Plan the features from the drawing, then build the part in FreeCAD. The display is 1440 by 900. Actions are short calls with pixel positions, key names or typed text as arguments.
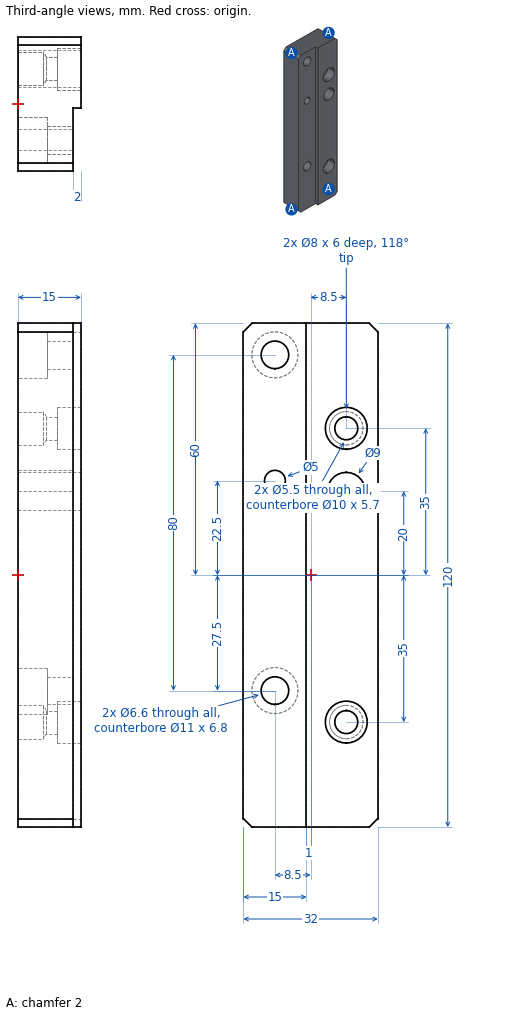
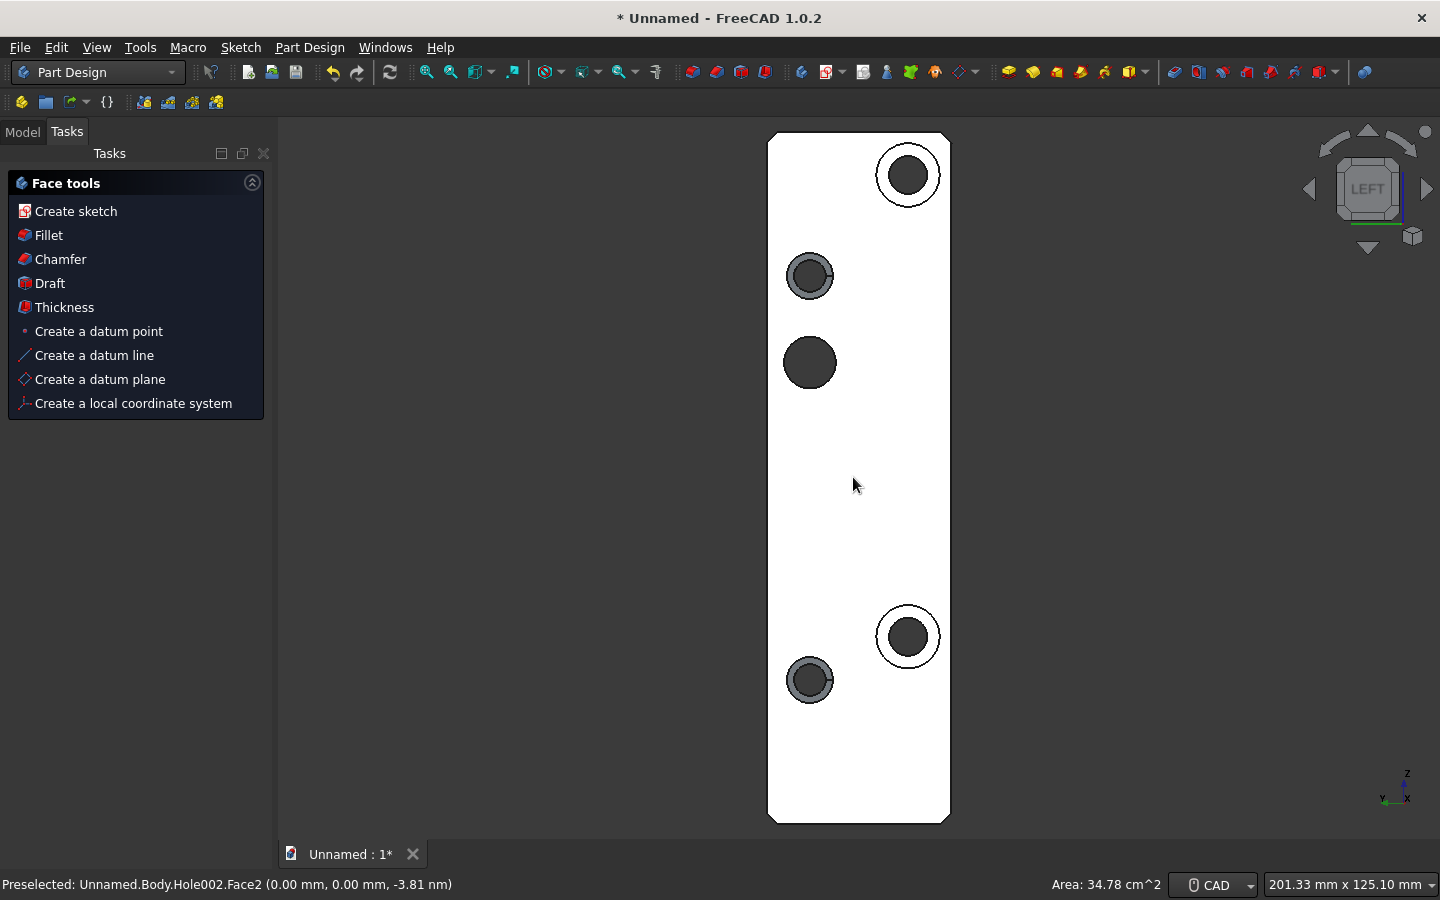
click(826, 72)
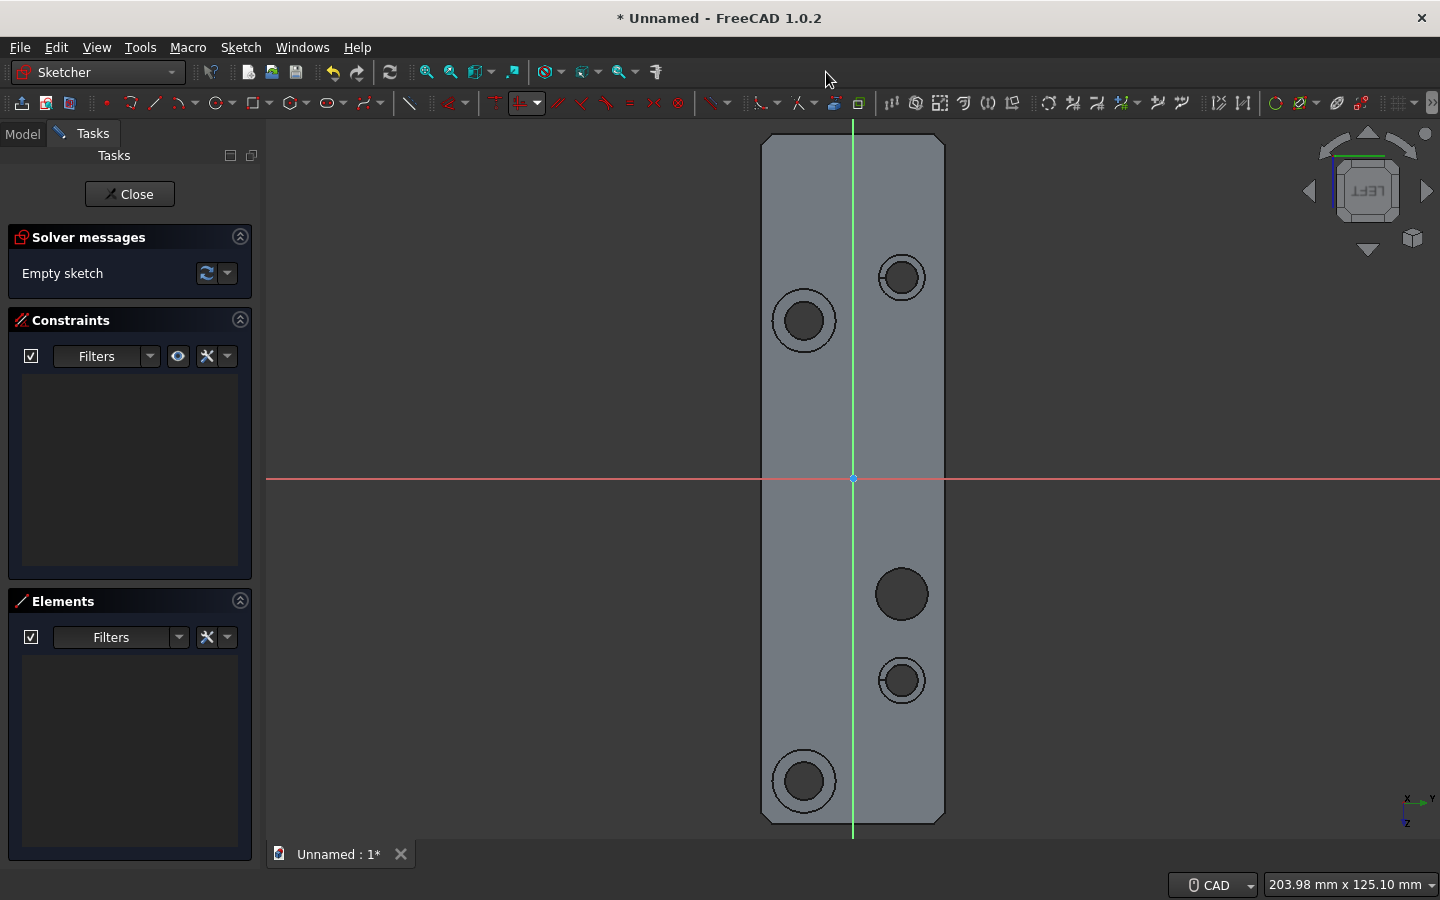
scroll(805, 617, up, 14)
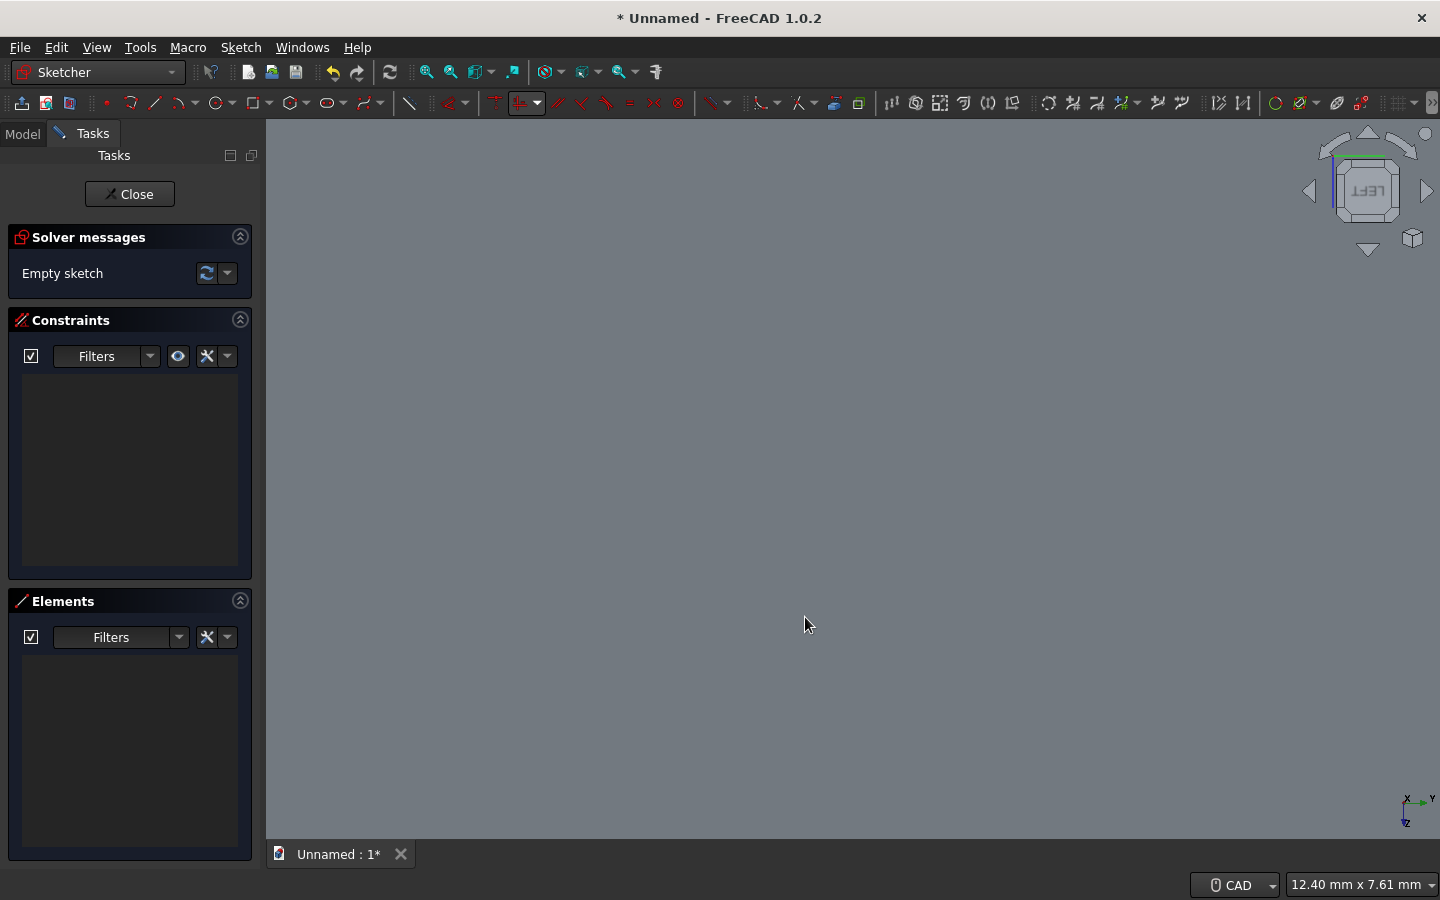
click(216, 104)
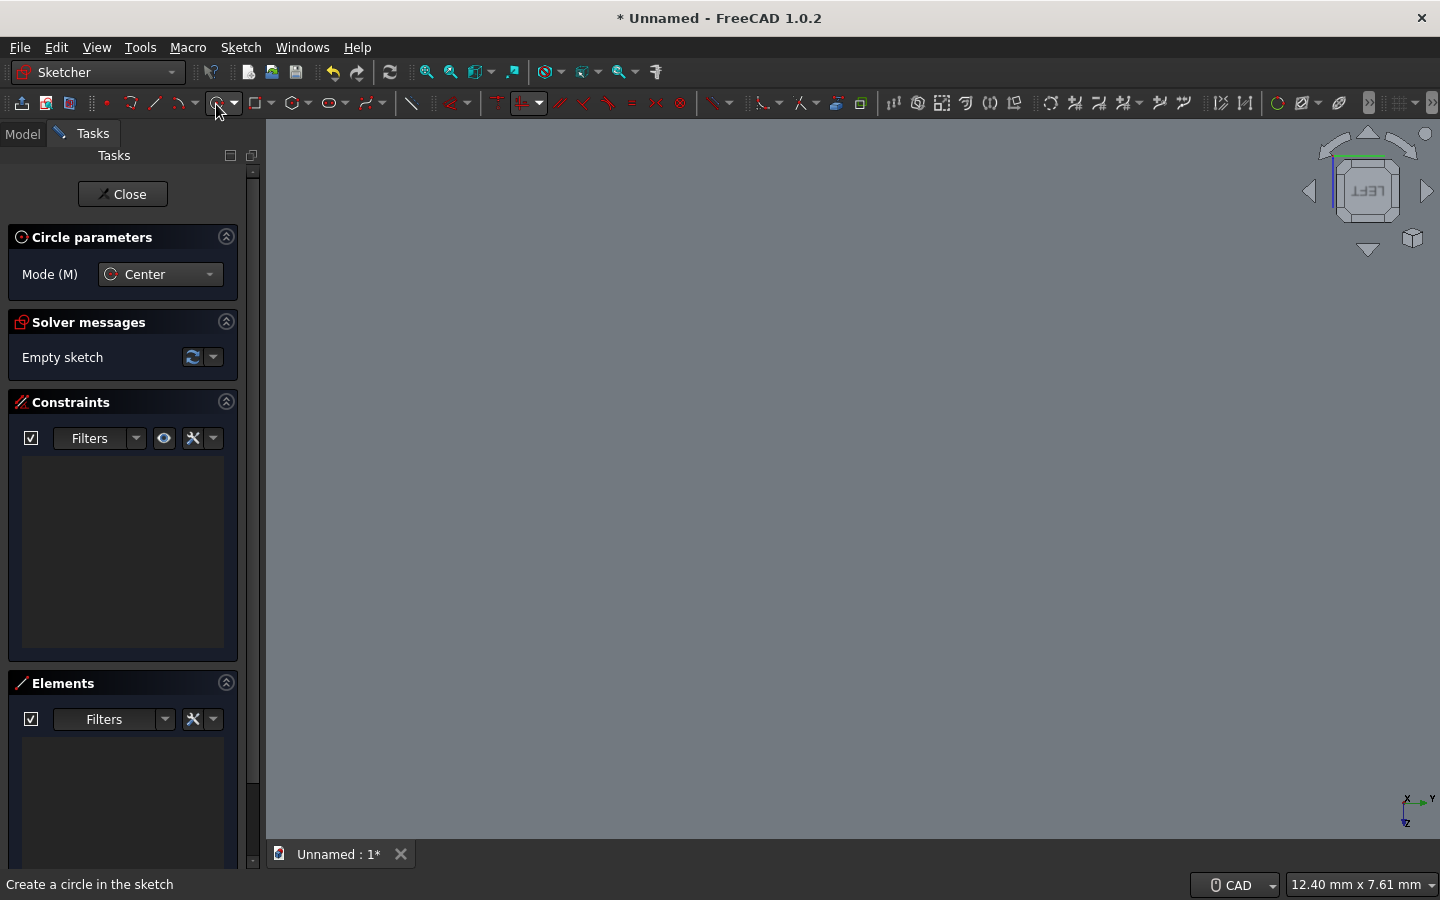
click(783, 467)
click(950, 299)
key(Escape)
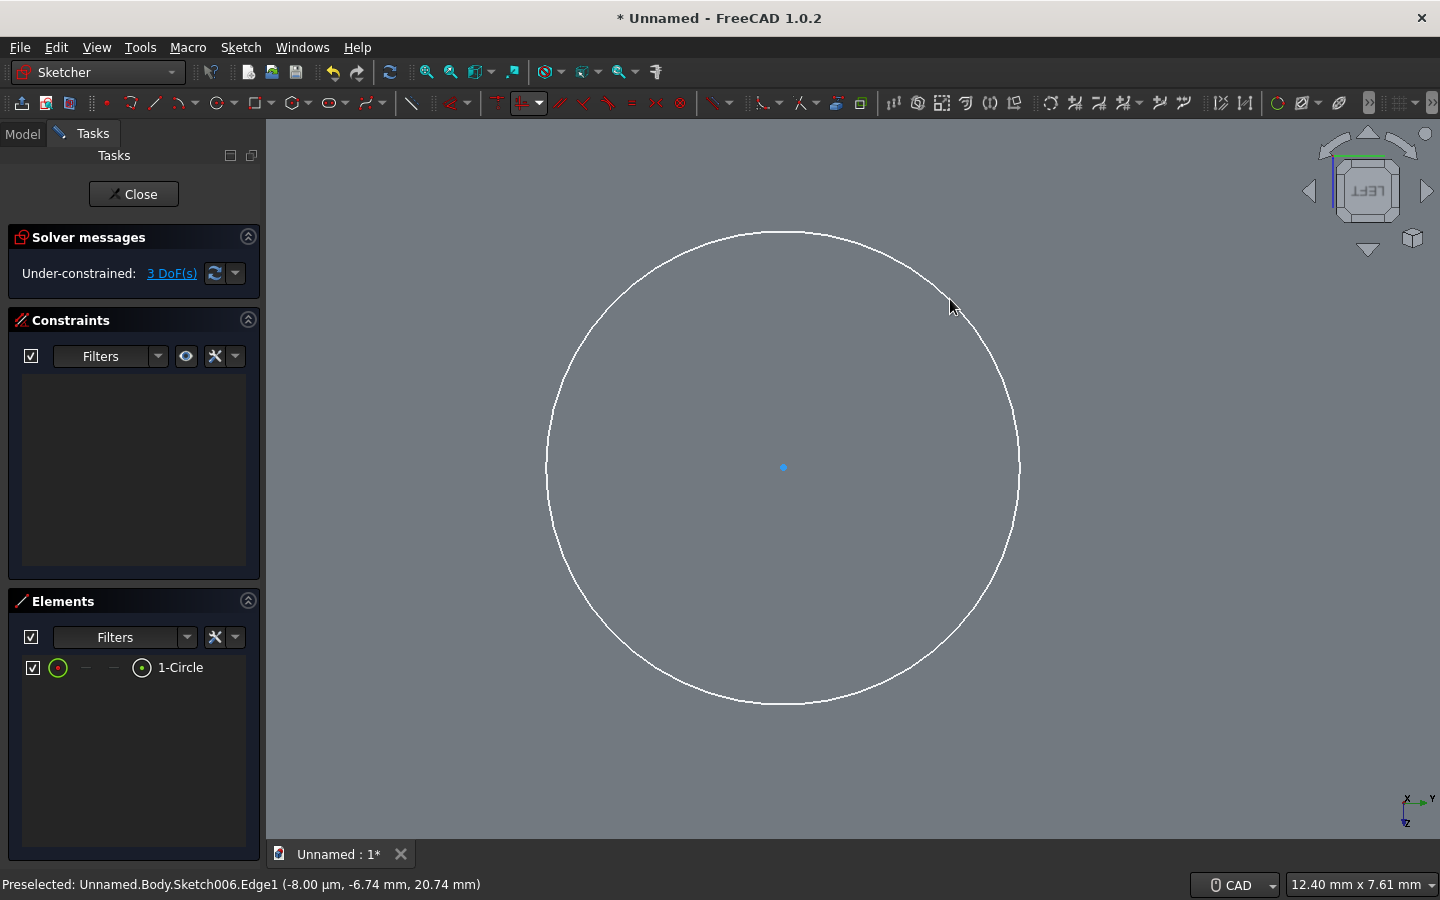
click(450, 104)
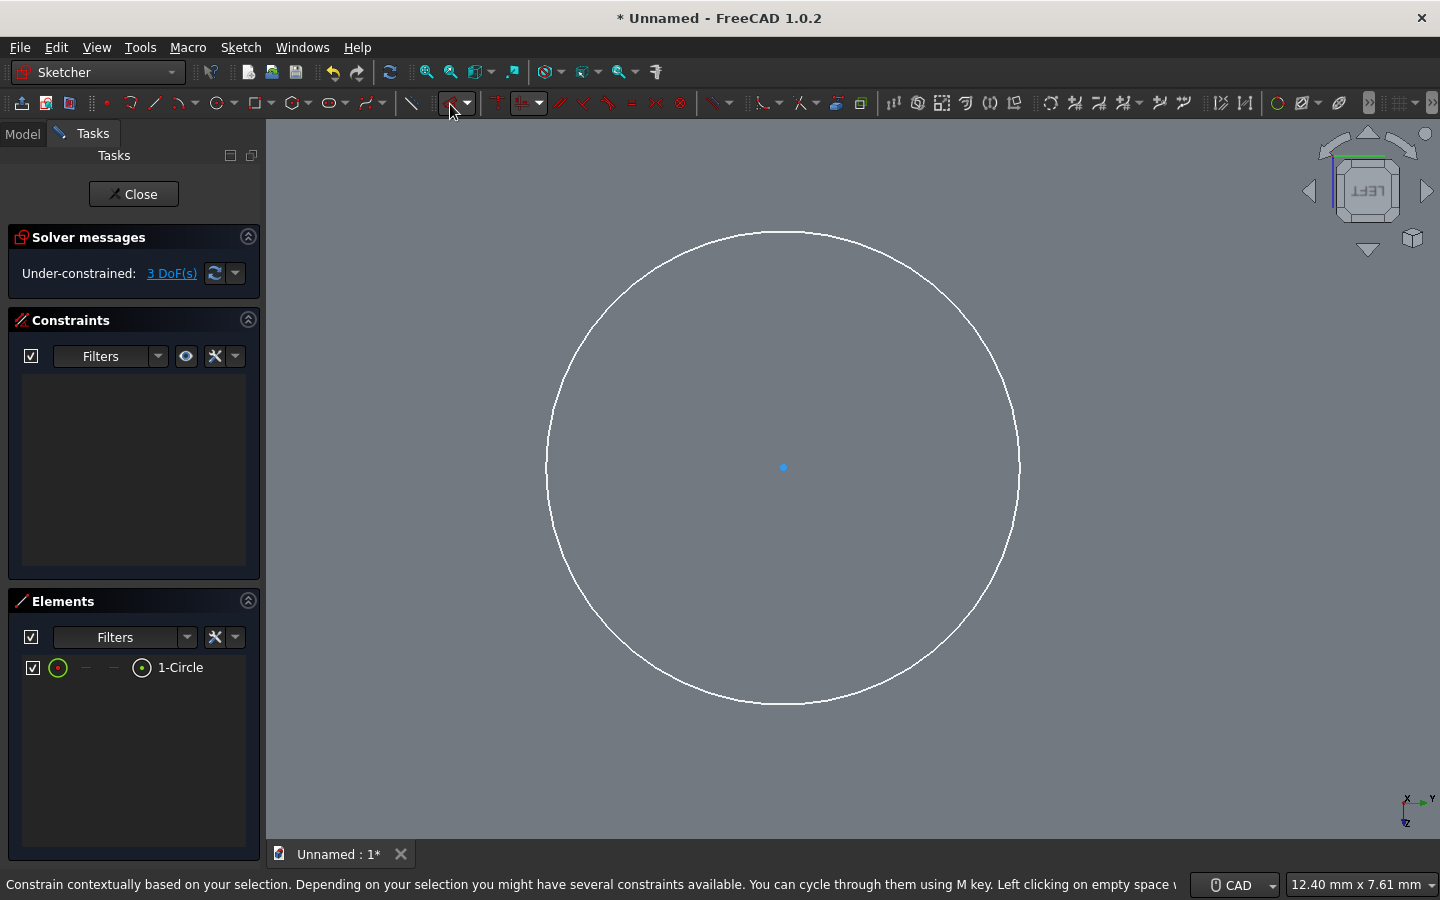
click(950, 300)
click(973, 277)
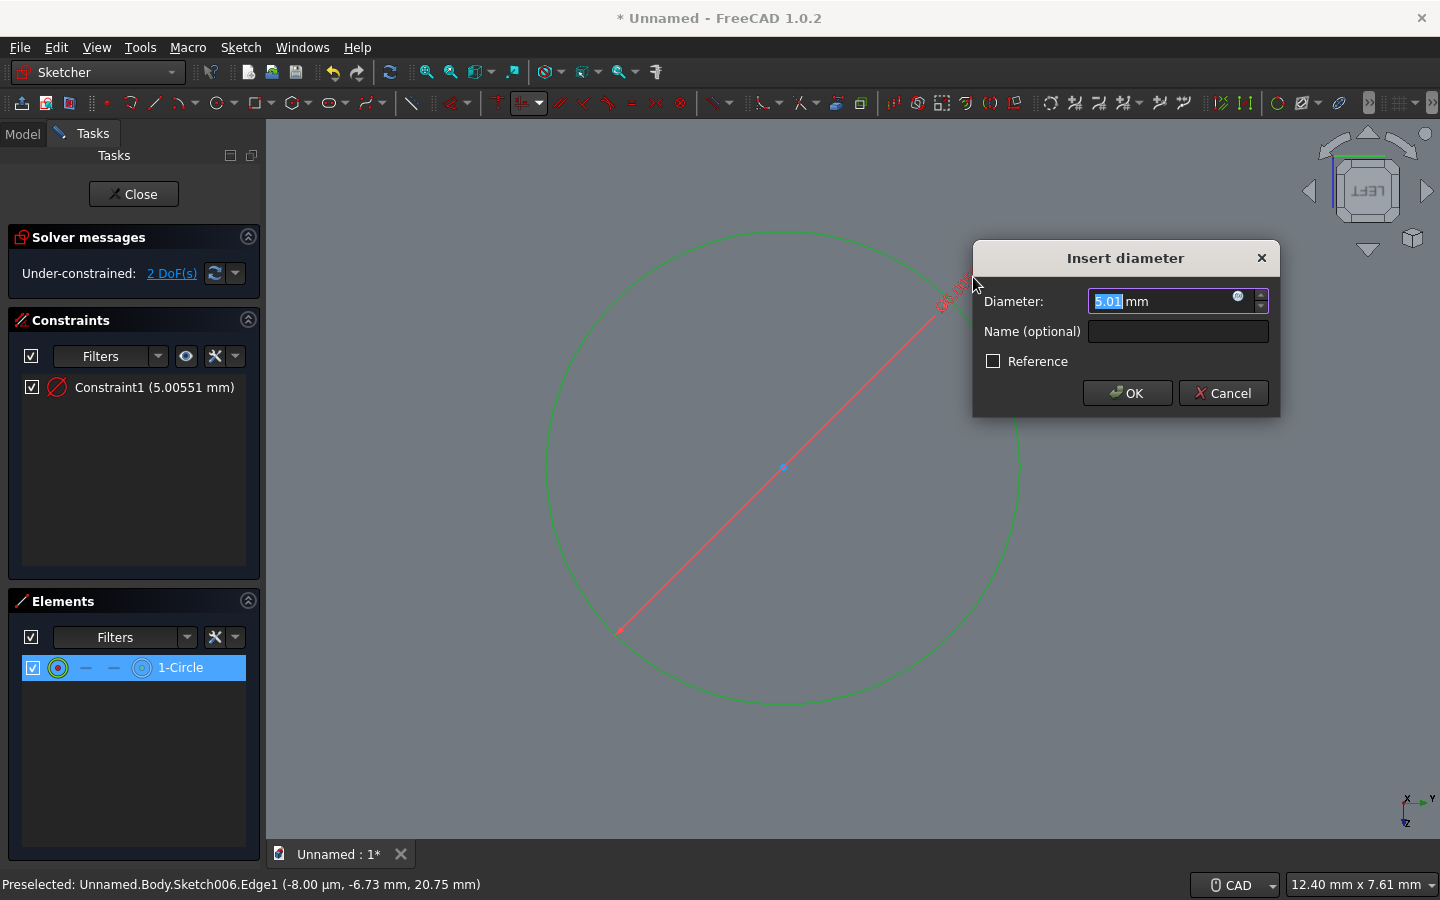
text(5)
key(Return)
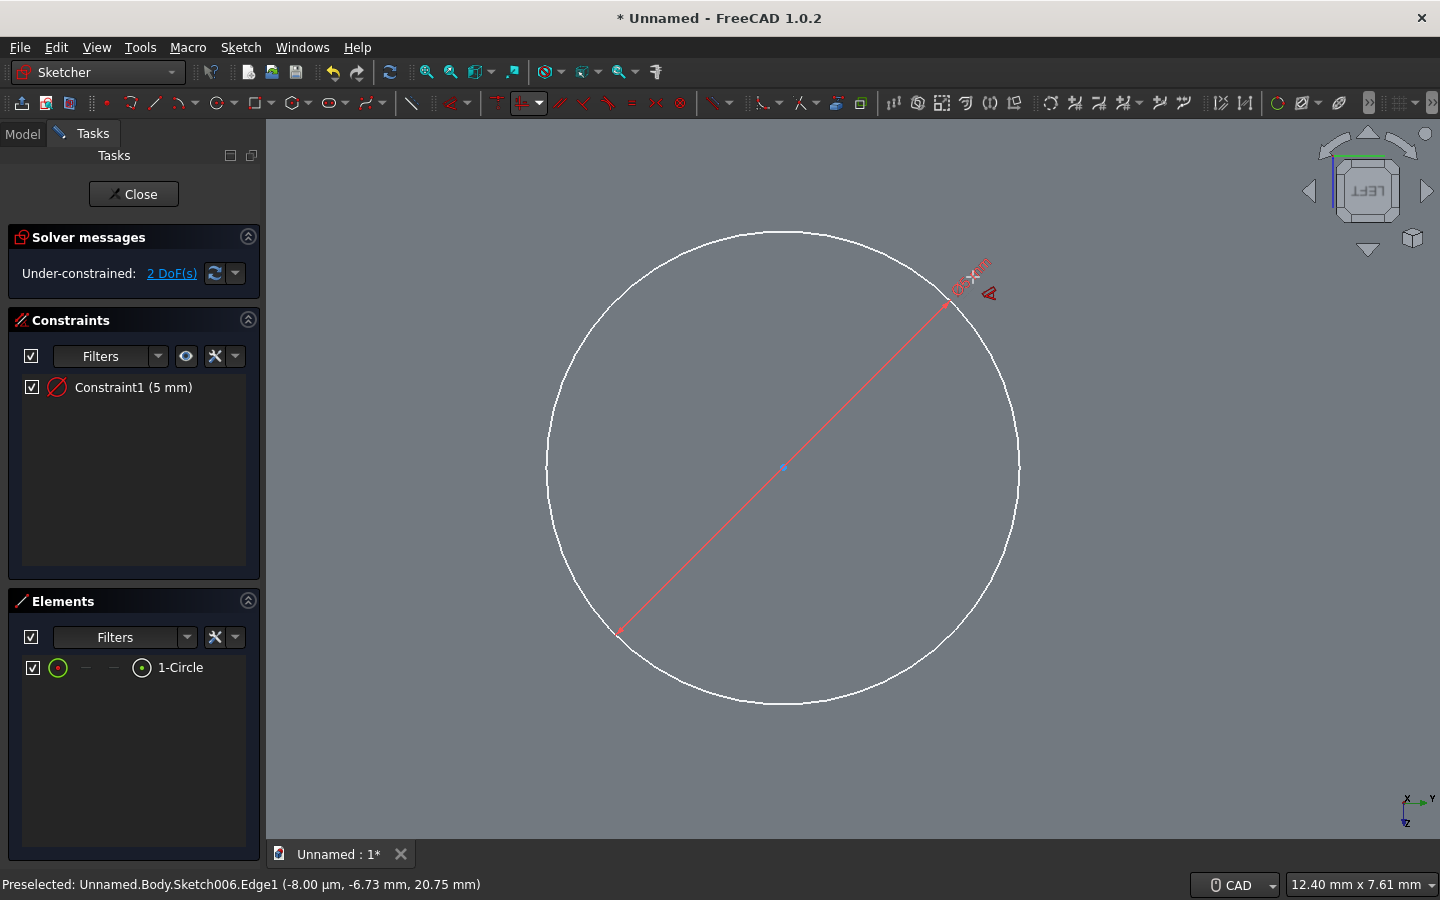
click(783, 468)
click(916, 502)